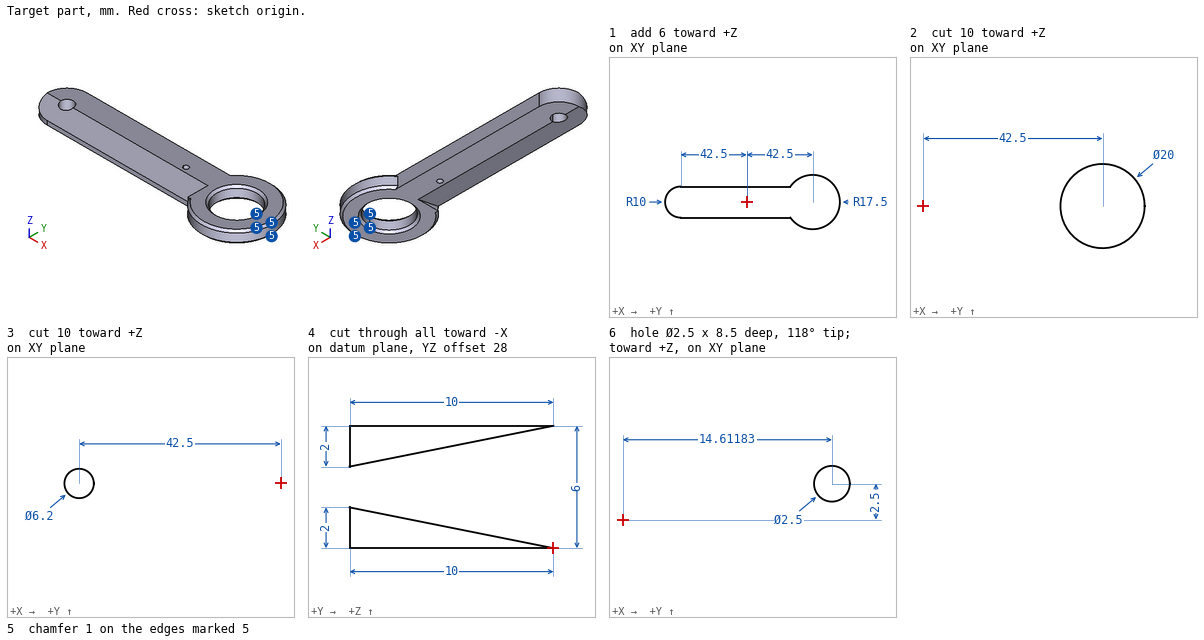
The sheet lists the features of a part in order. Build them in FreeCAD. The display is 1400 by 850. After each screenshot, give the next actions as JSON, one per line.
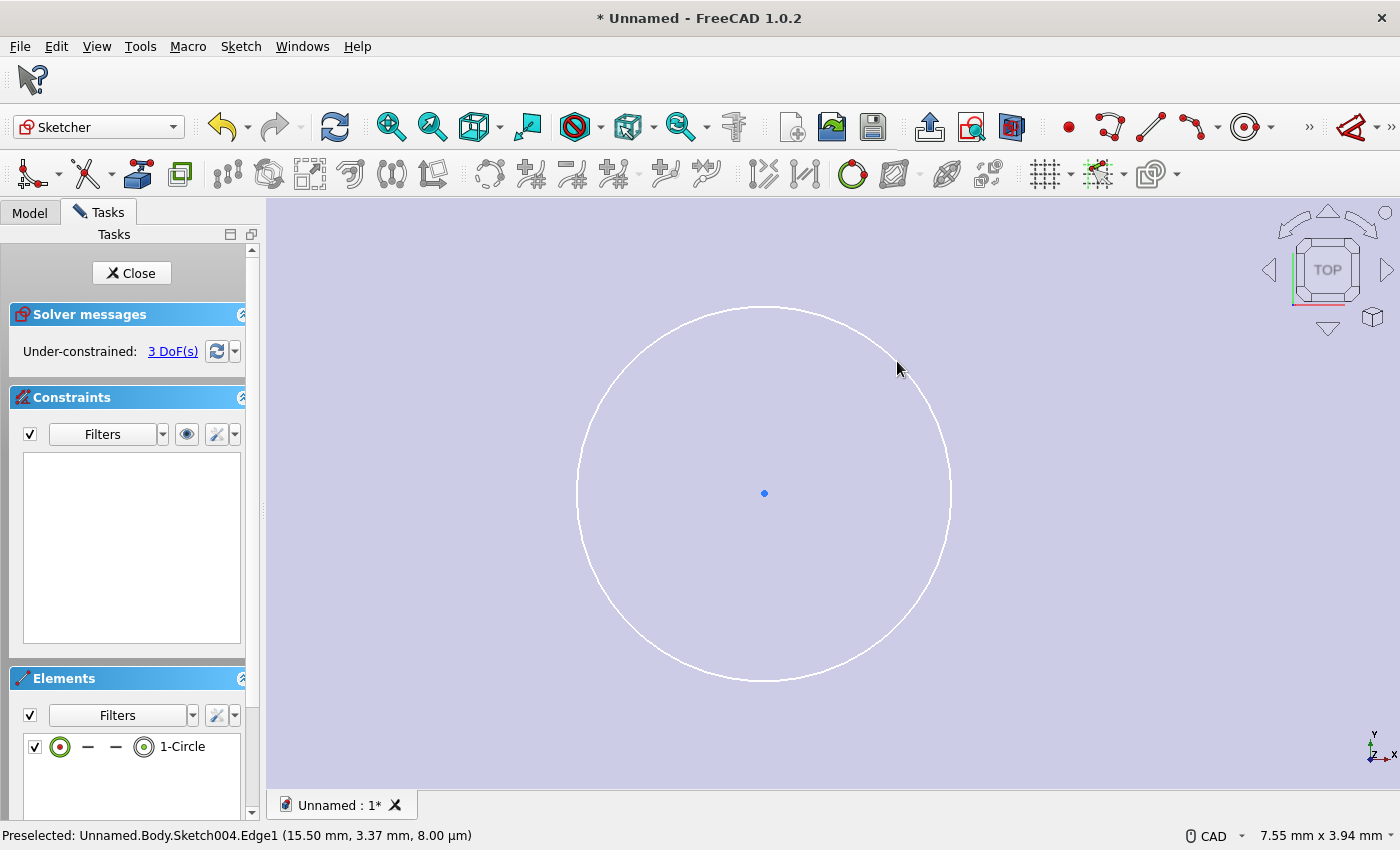
{"action": "key", "text": "d"}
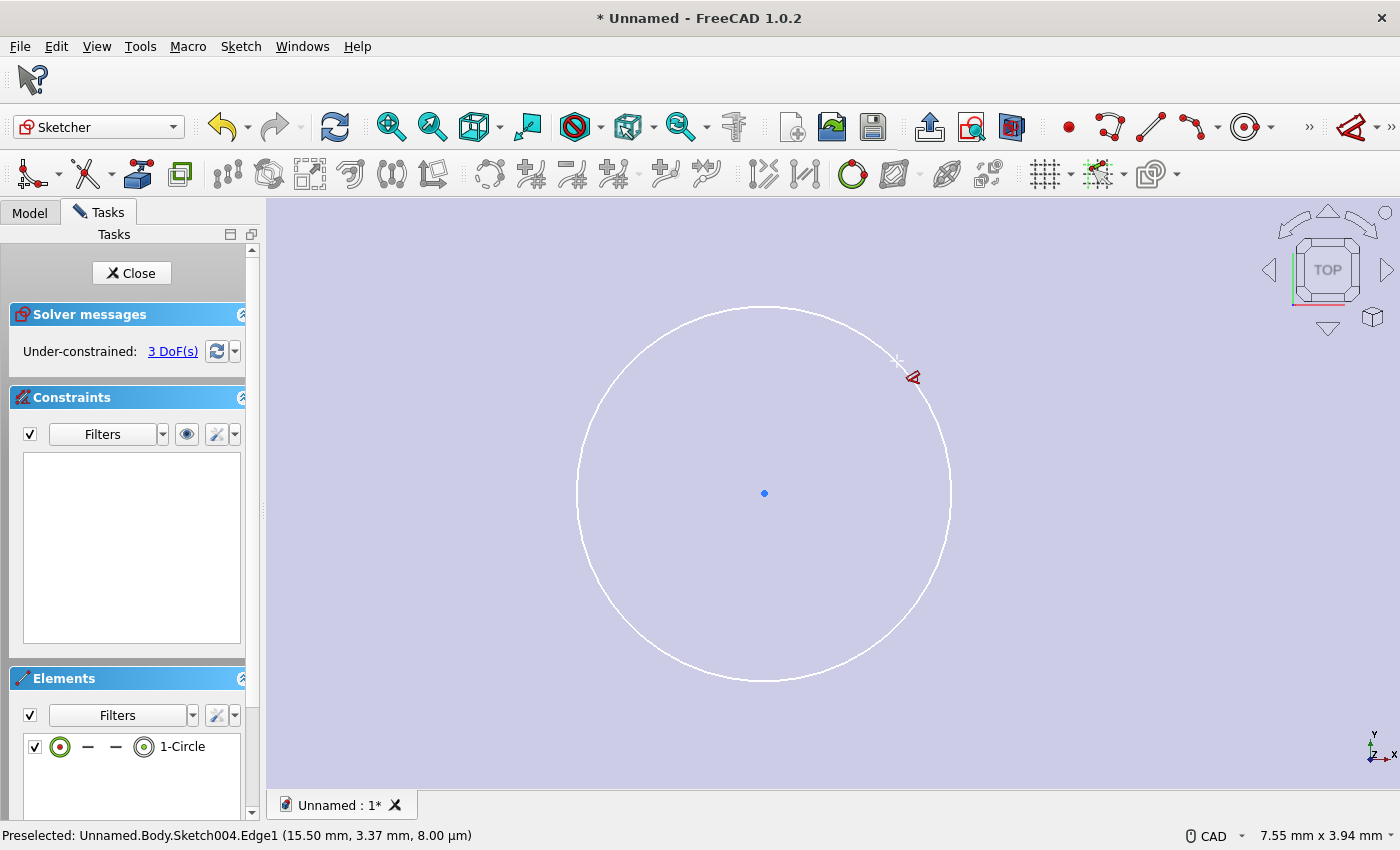
{"action": "left_click", "coordinate": [896, 361]}
{"action": "left_click", "coordinate": [919, 338]}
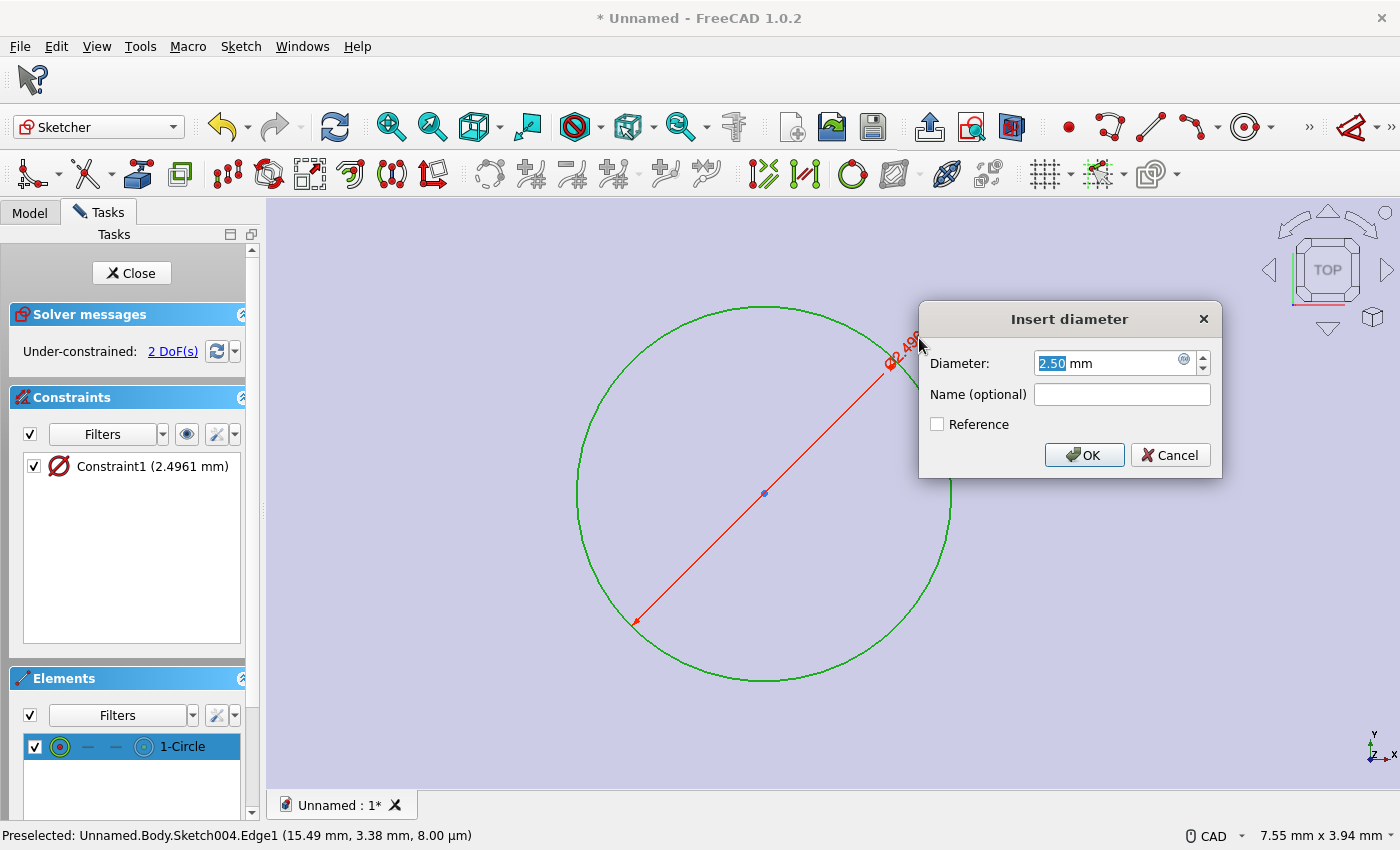
{"action": "type", "text": "2.5"}
{"action": "key", "text": "Return"}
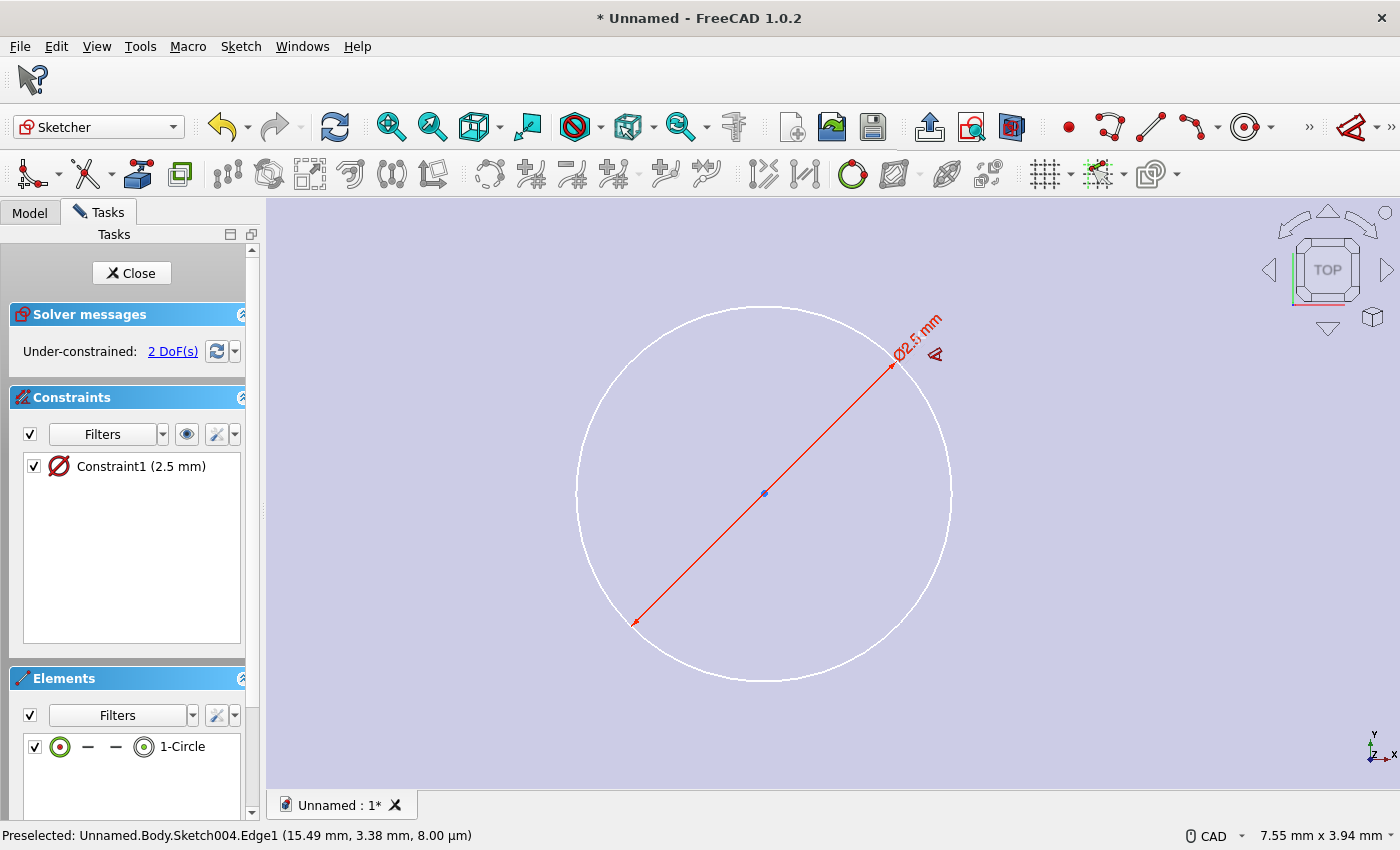
{"action": "left_click", "coordinate": [764, 494]}
{"action": "left_click", "coordinate": [798, 627]}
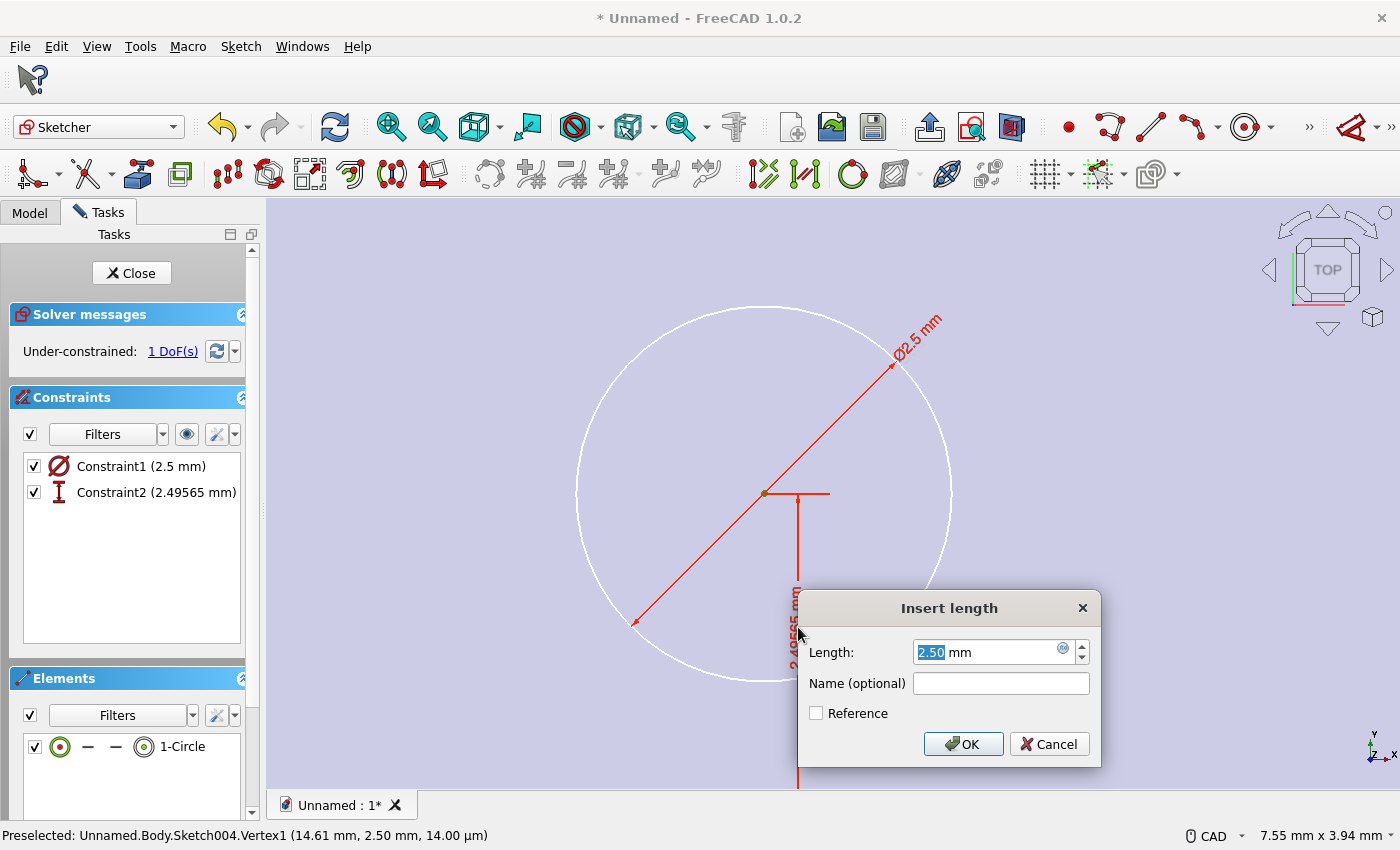
{"action": "type", "text": "2.5"}
{"action": "key", "text": "Return"}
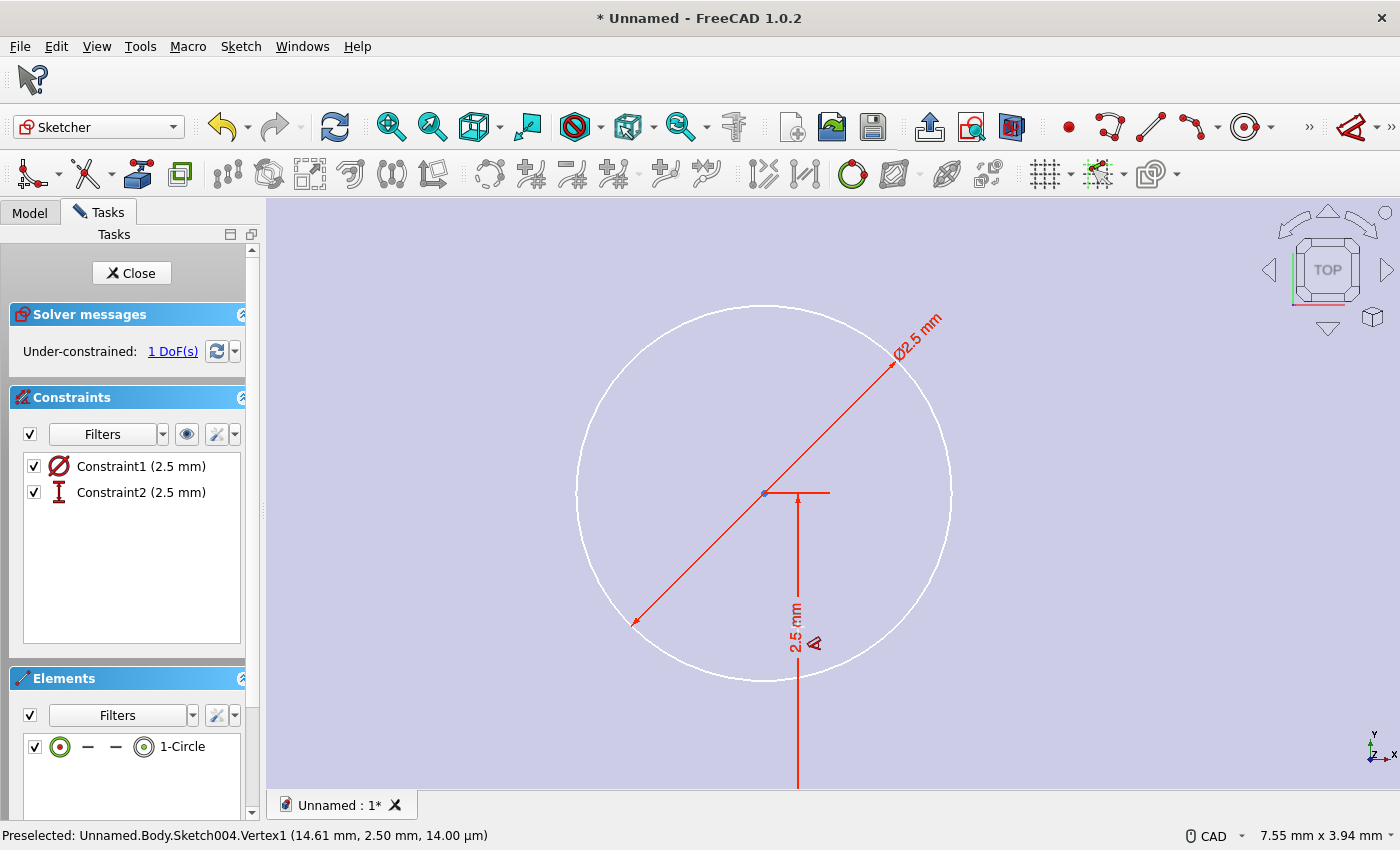
{"action": "left_click", "coordinate": [764, 493]}
{"action": "left_click", "coordinate": [529, 459]}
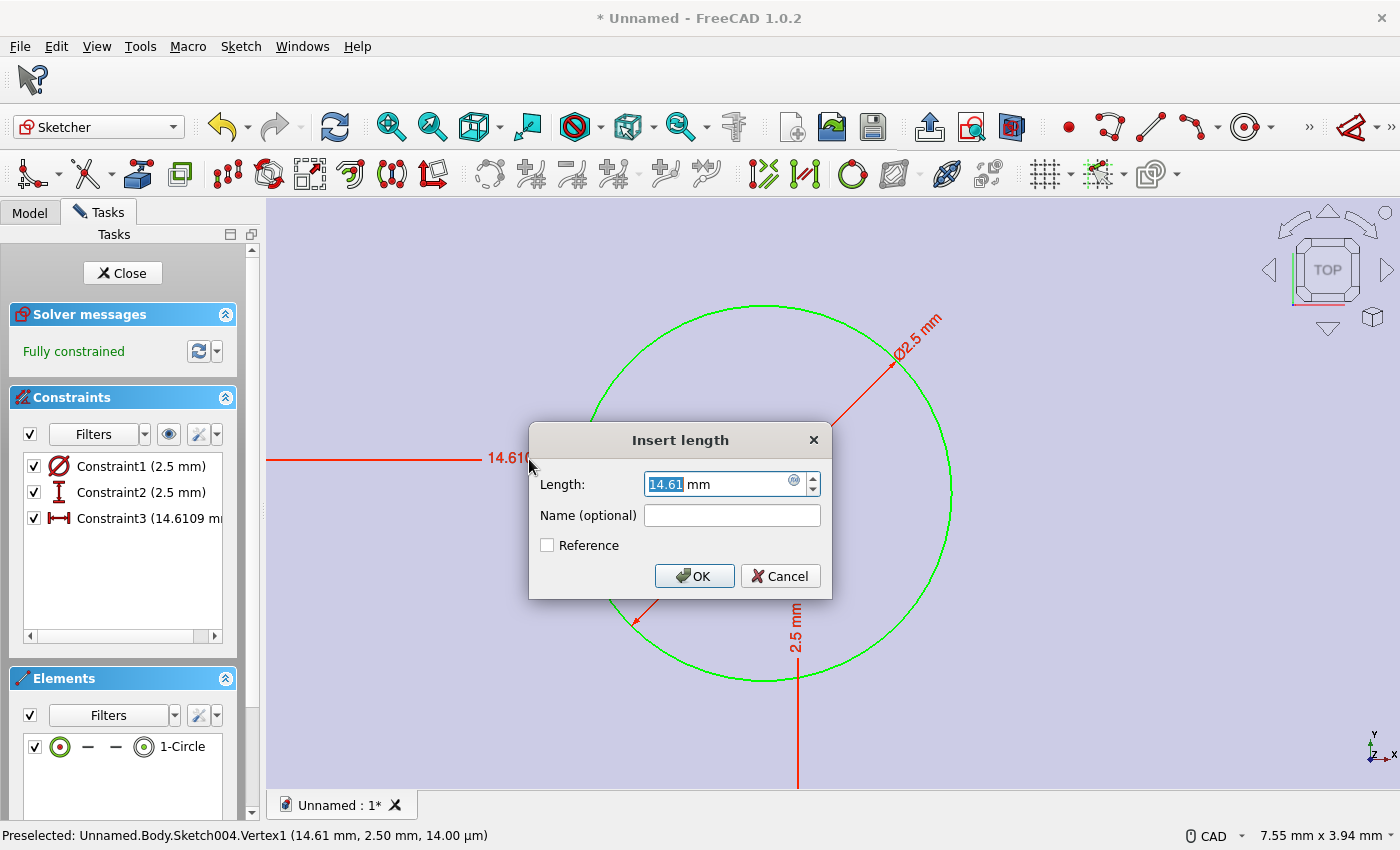
{"action": "type", "text": "14.61183"}
{"action": "key", "text": "Return"}
{"action": "key", "text": "Escape"}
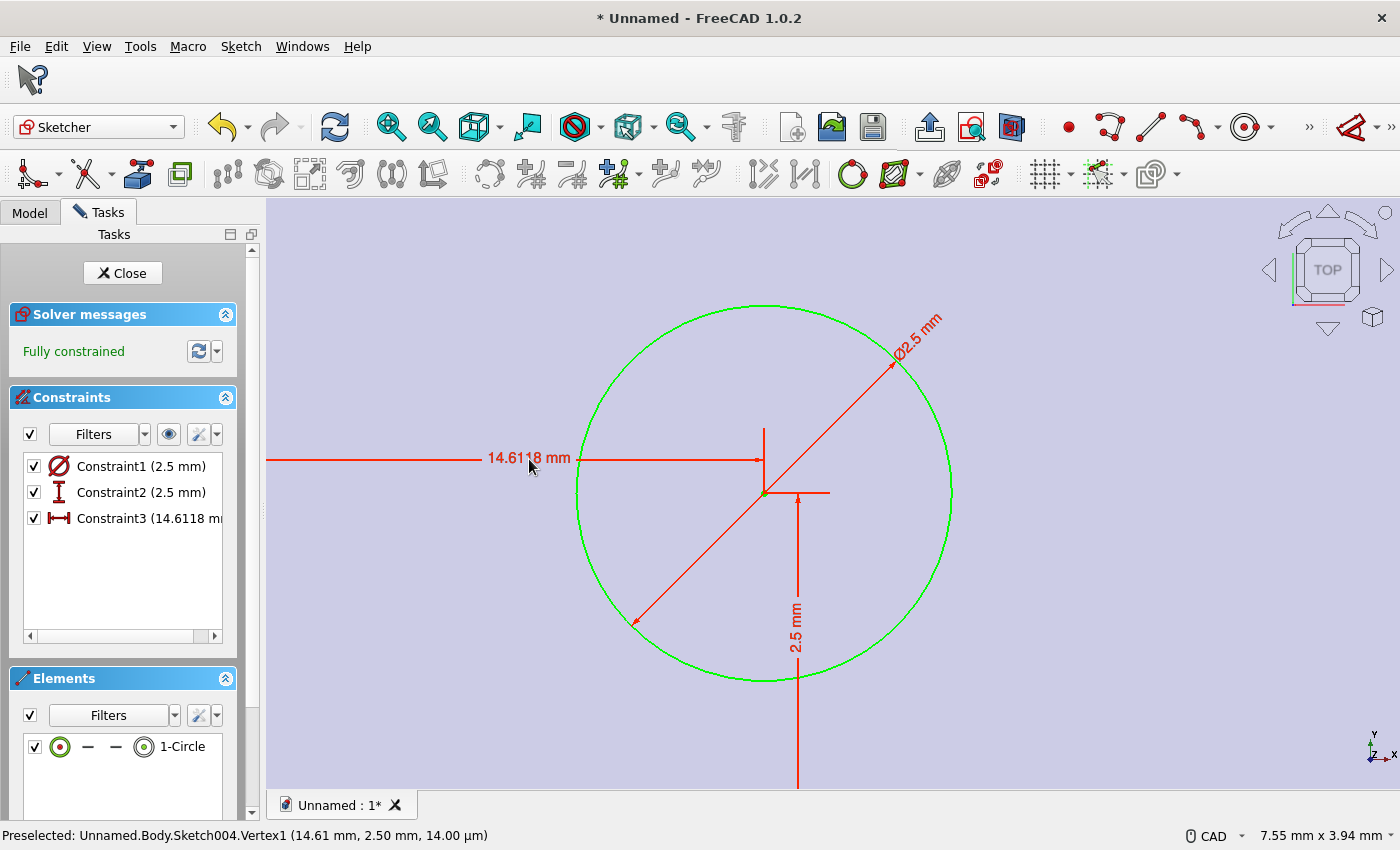
{"action": "left_click", "coordinate": [123, 273]}